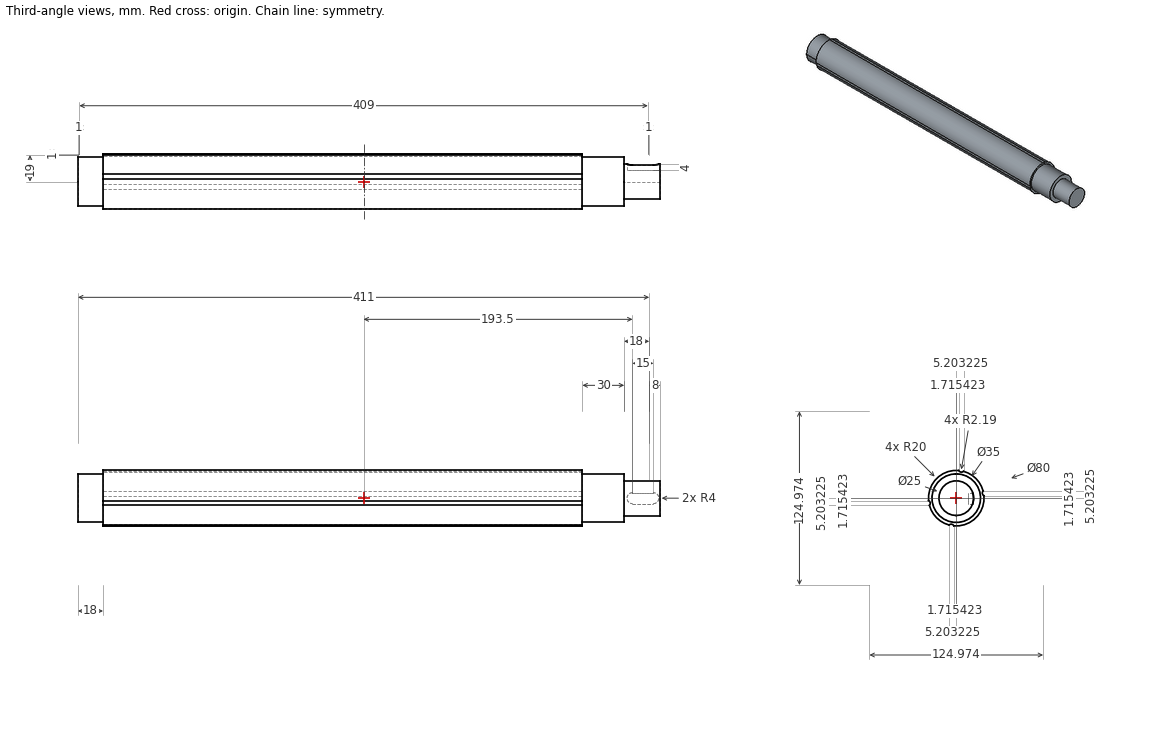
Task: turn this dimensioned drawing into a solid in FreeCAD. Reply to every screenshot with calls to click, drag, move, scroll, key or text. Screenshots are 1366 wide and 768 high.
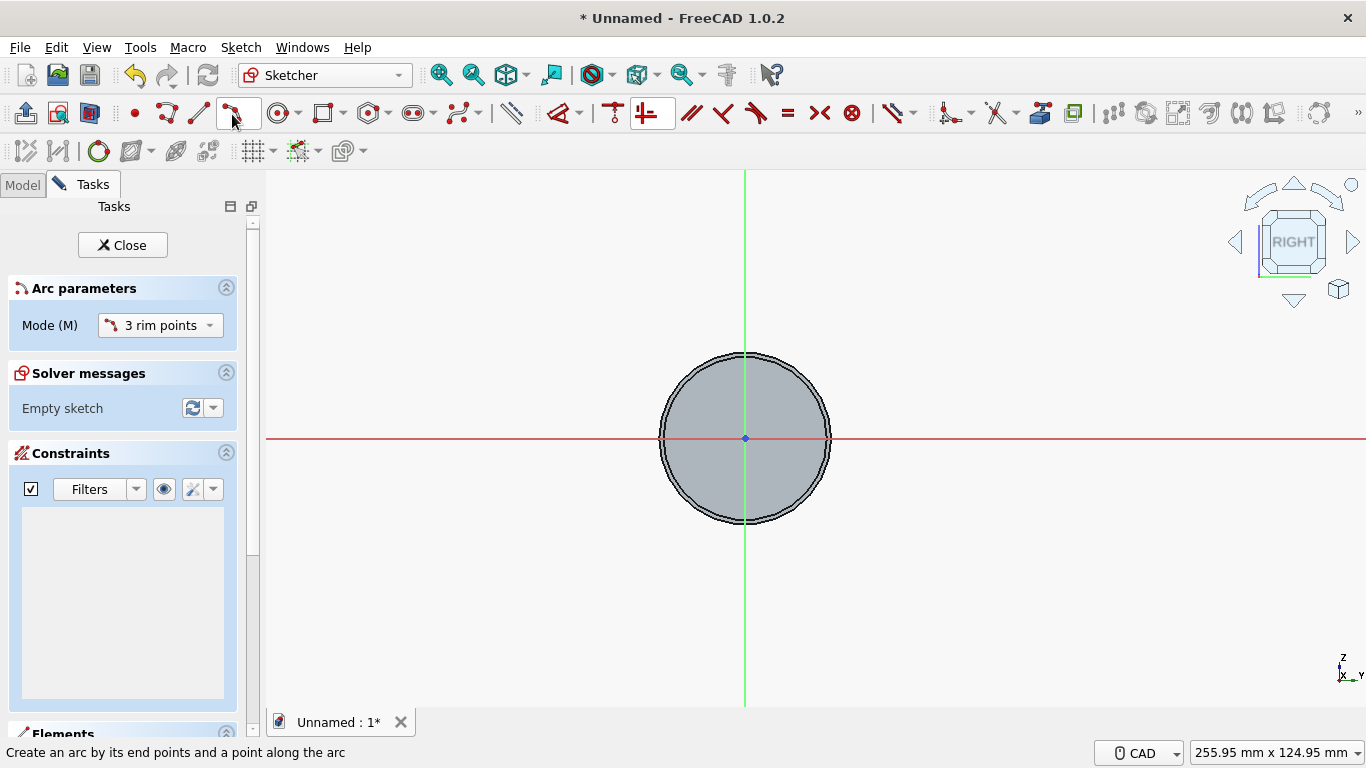
click(768, 356)
click(828, 416)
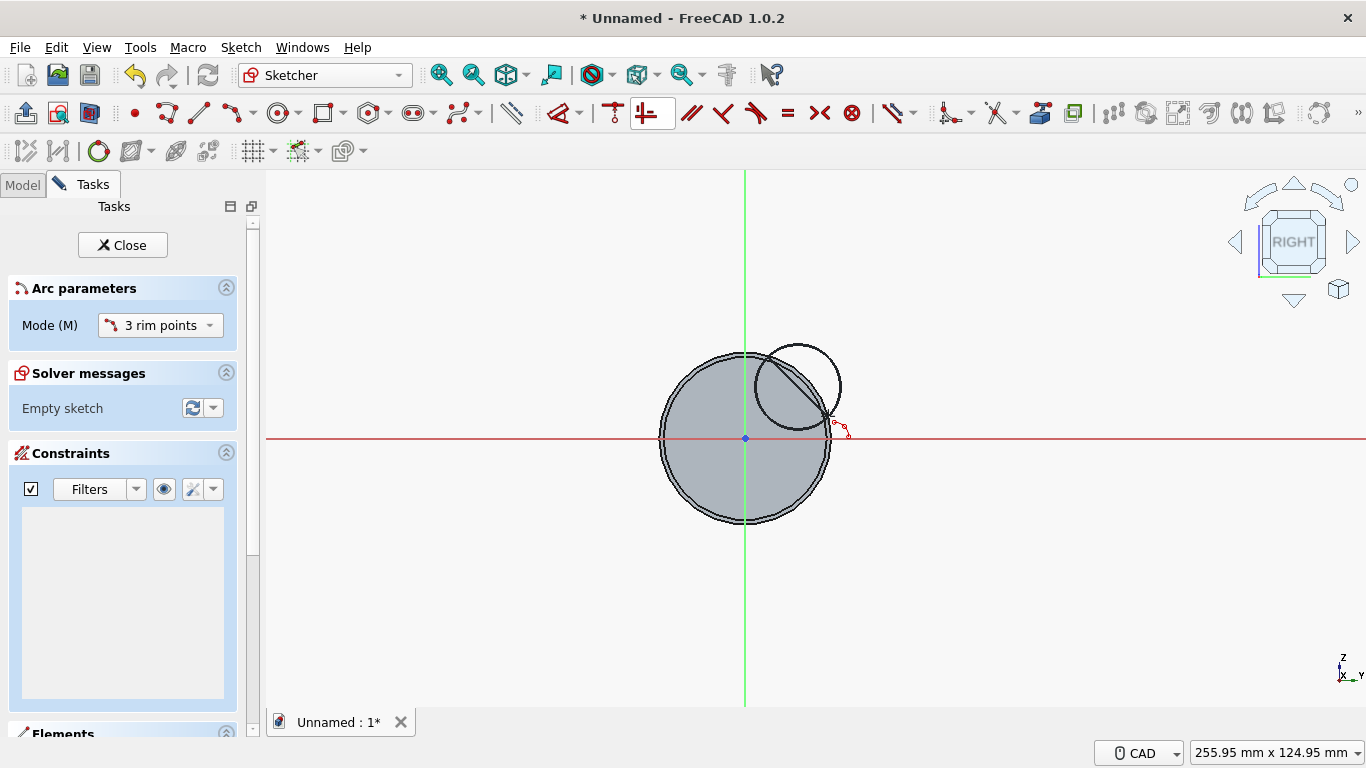
scroll(806, 378, up, 2)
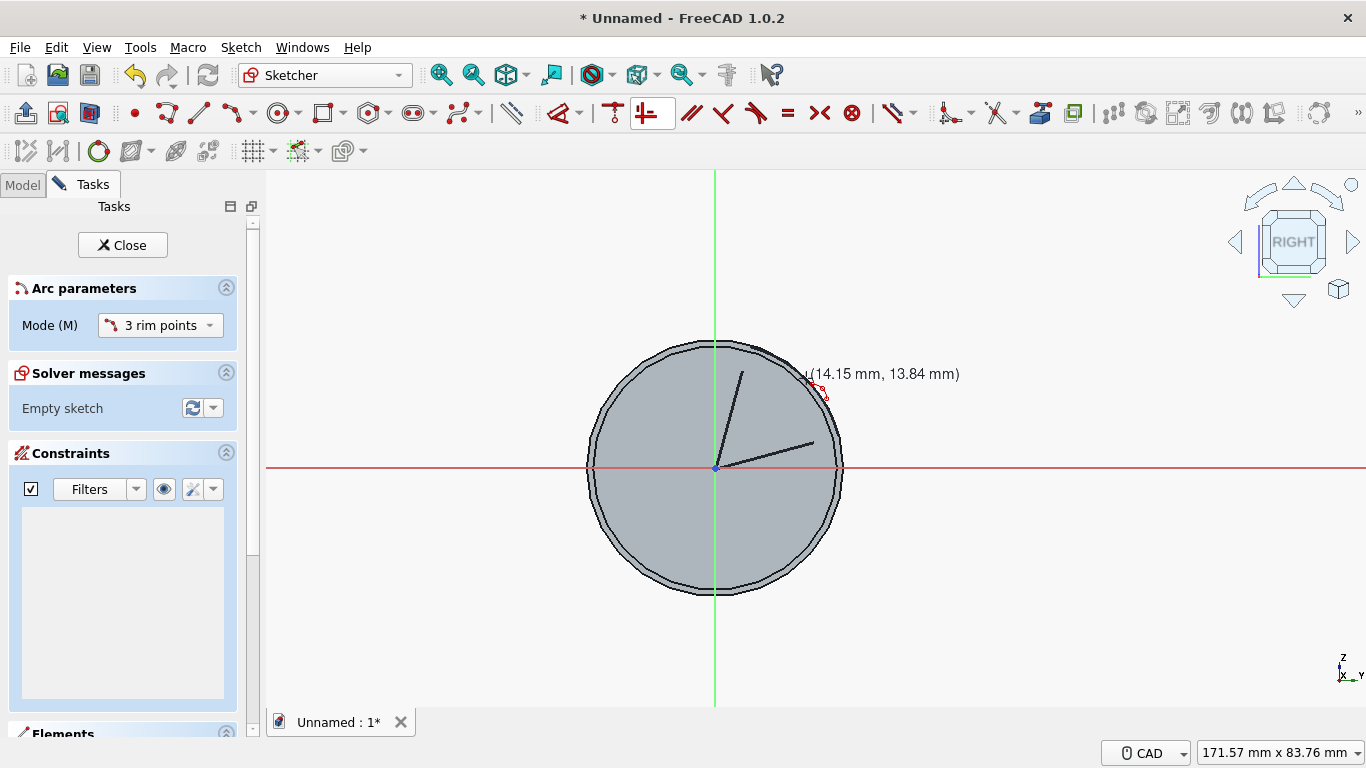
click(806, 377)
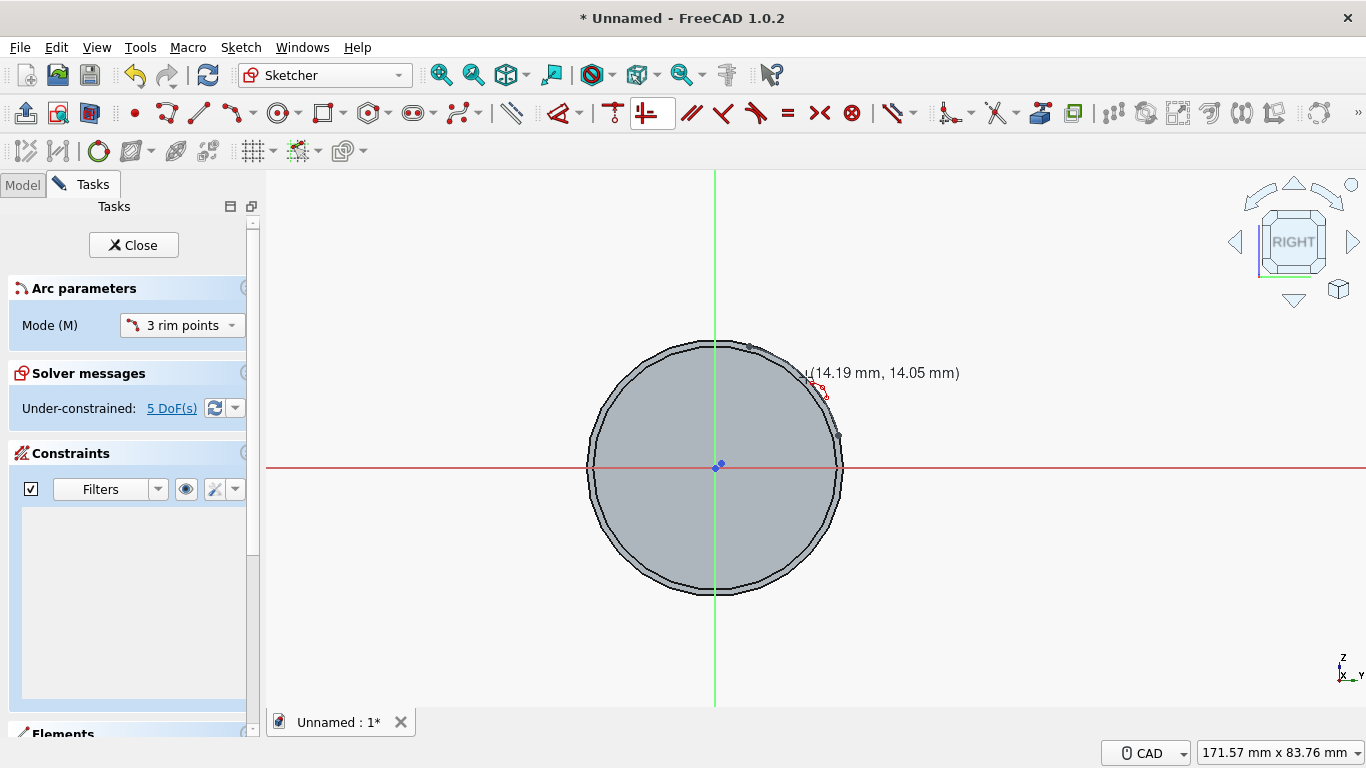
click(839, 436)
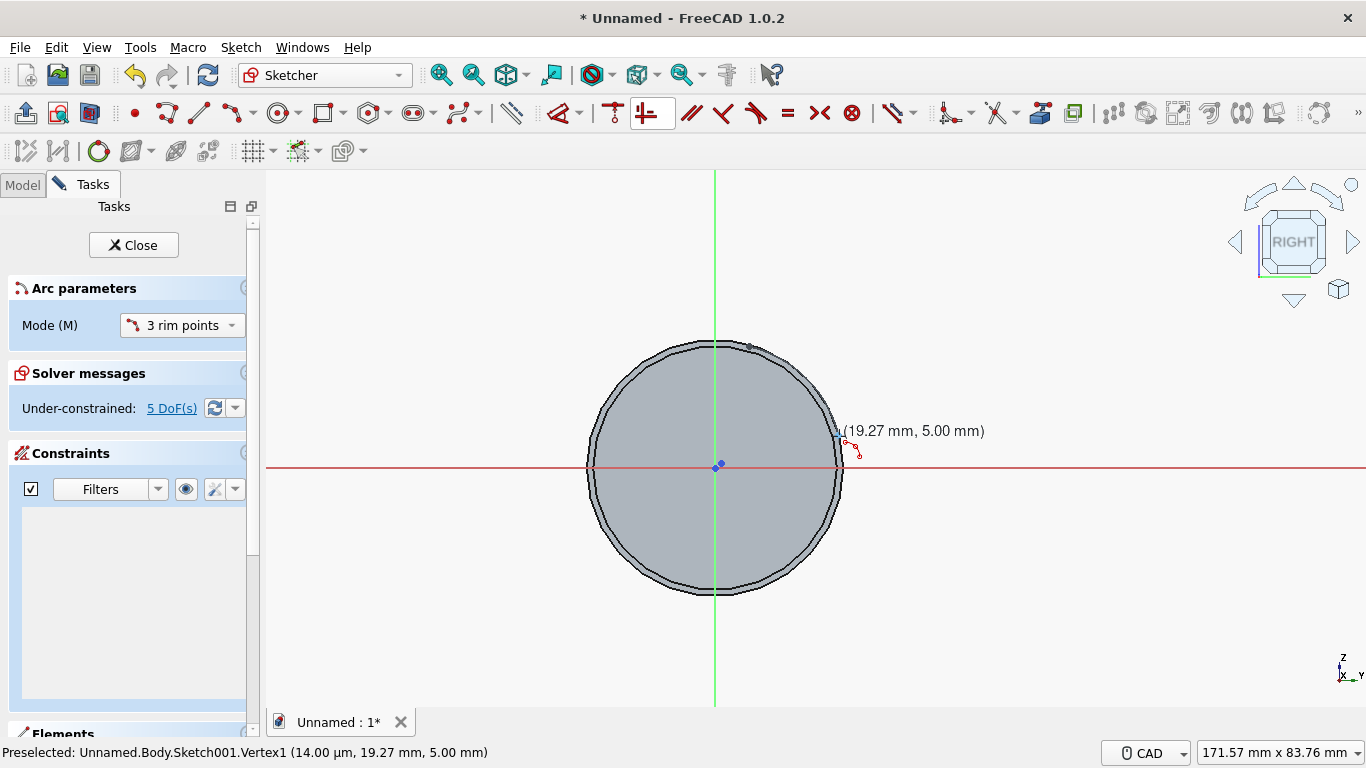
scroll(843, 457, up, 2)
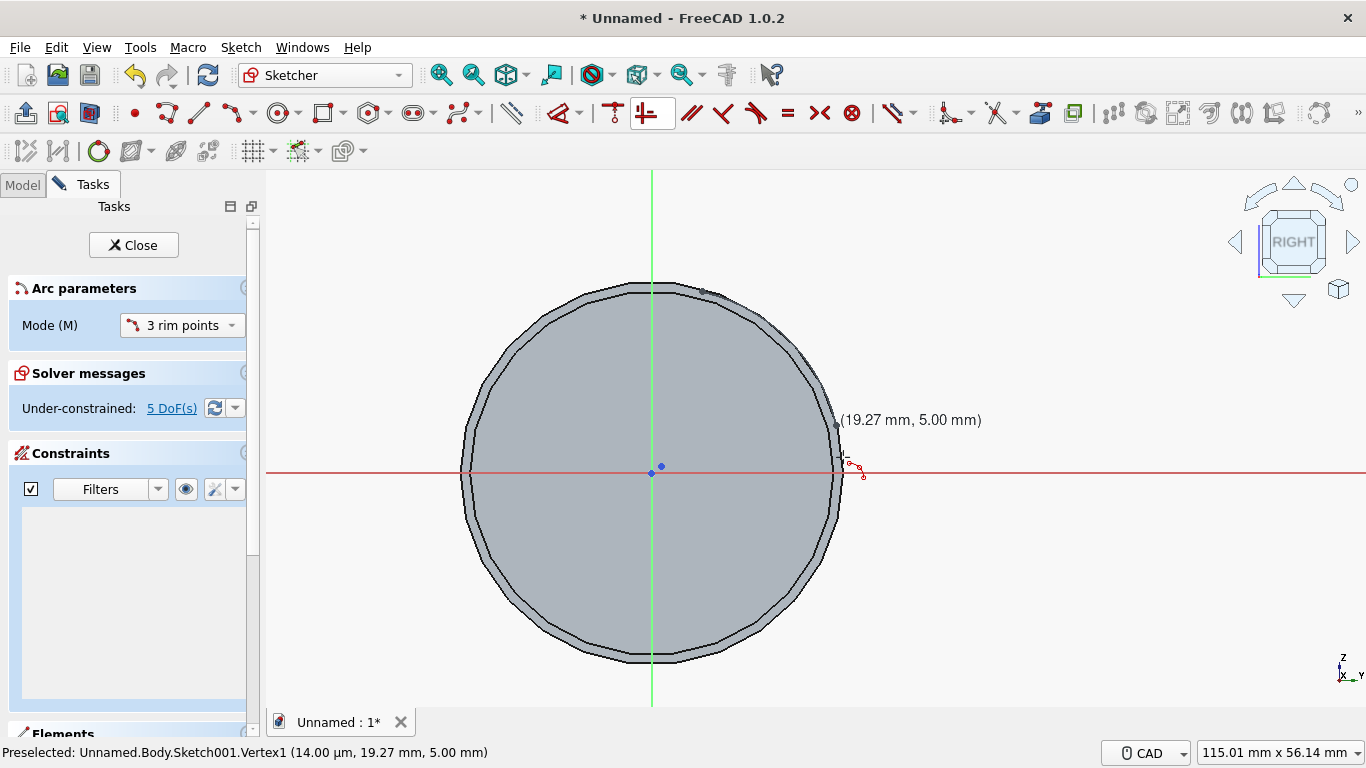
click(842, 457)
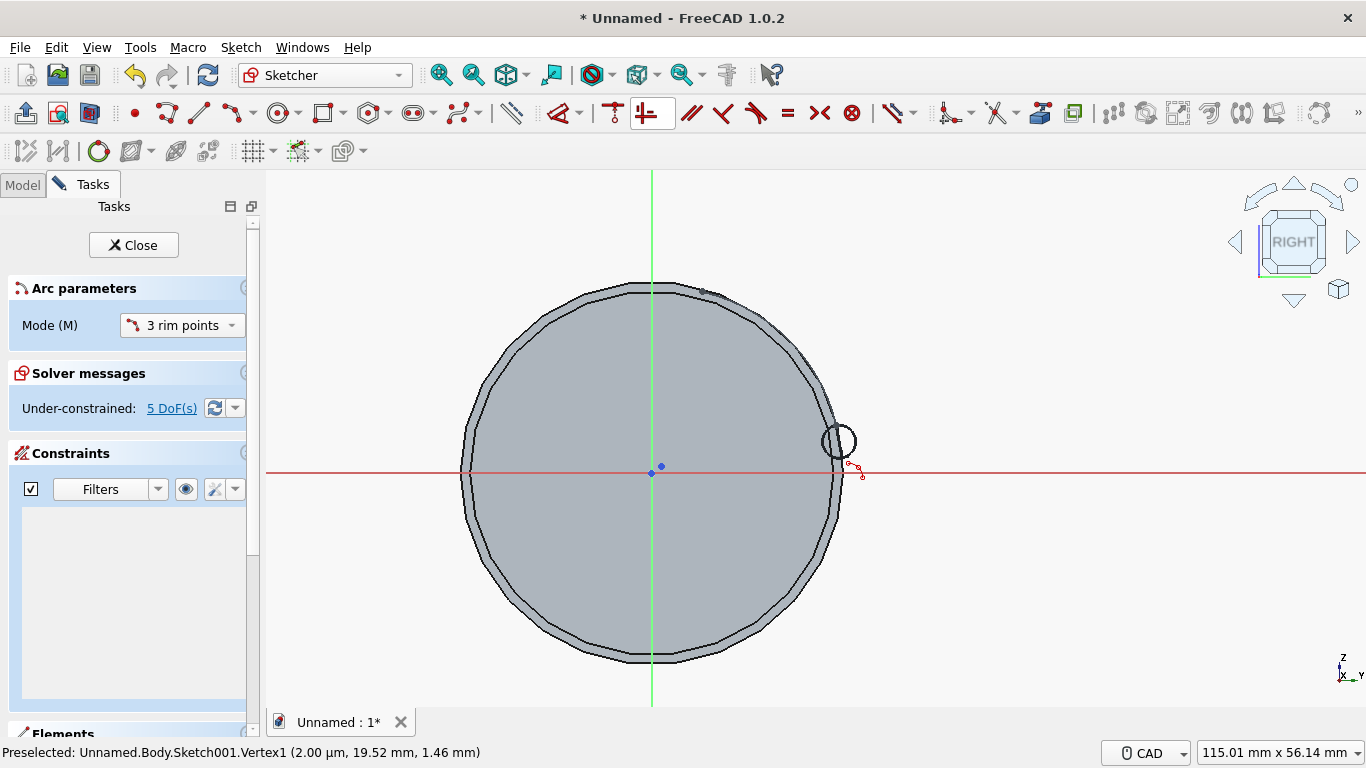
scroll(831, 442, up, 4)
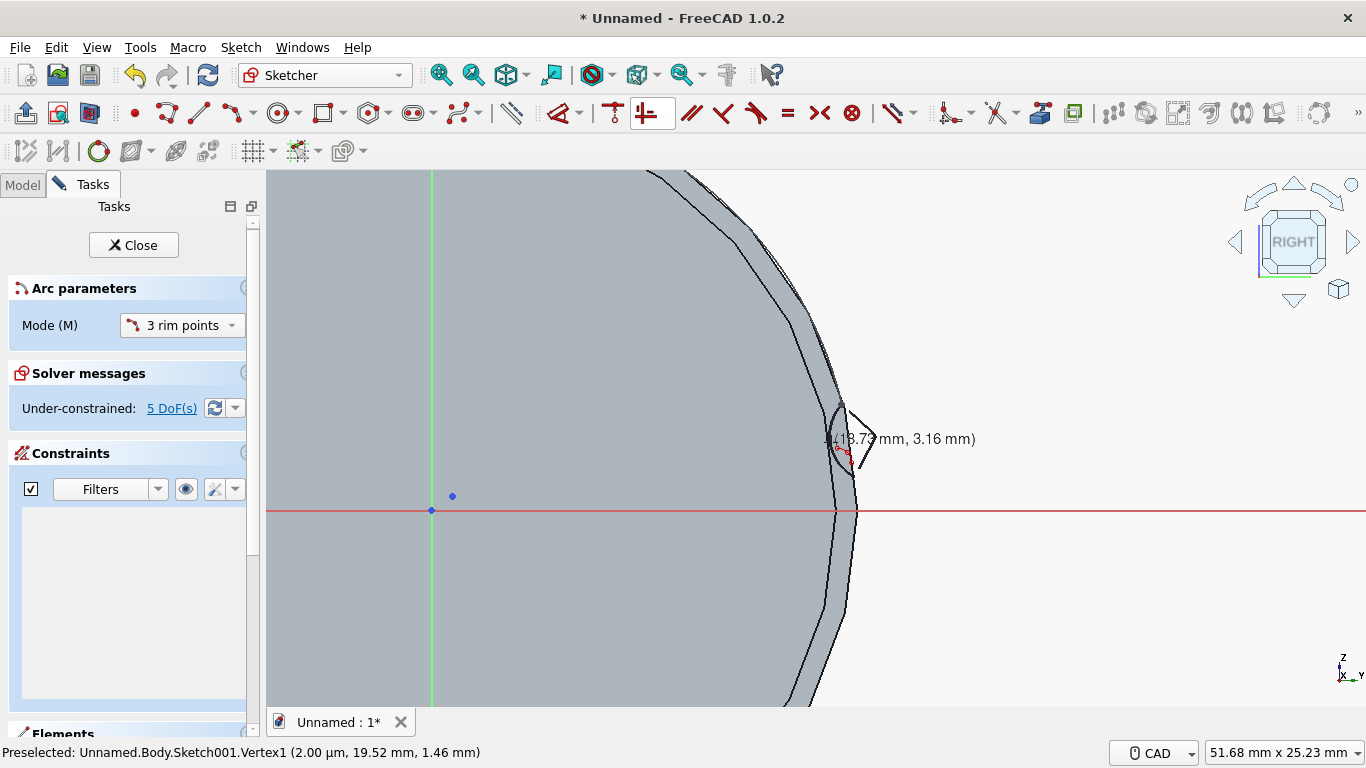
click(830, 441)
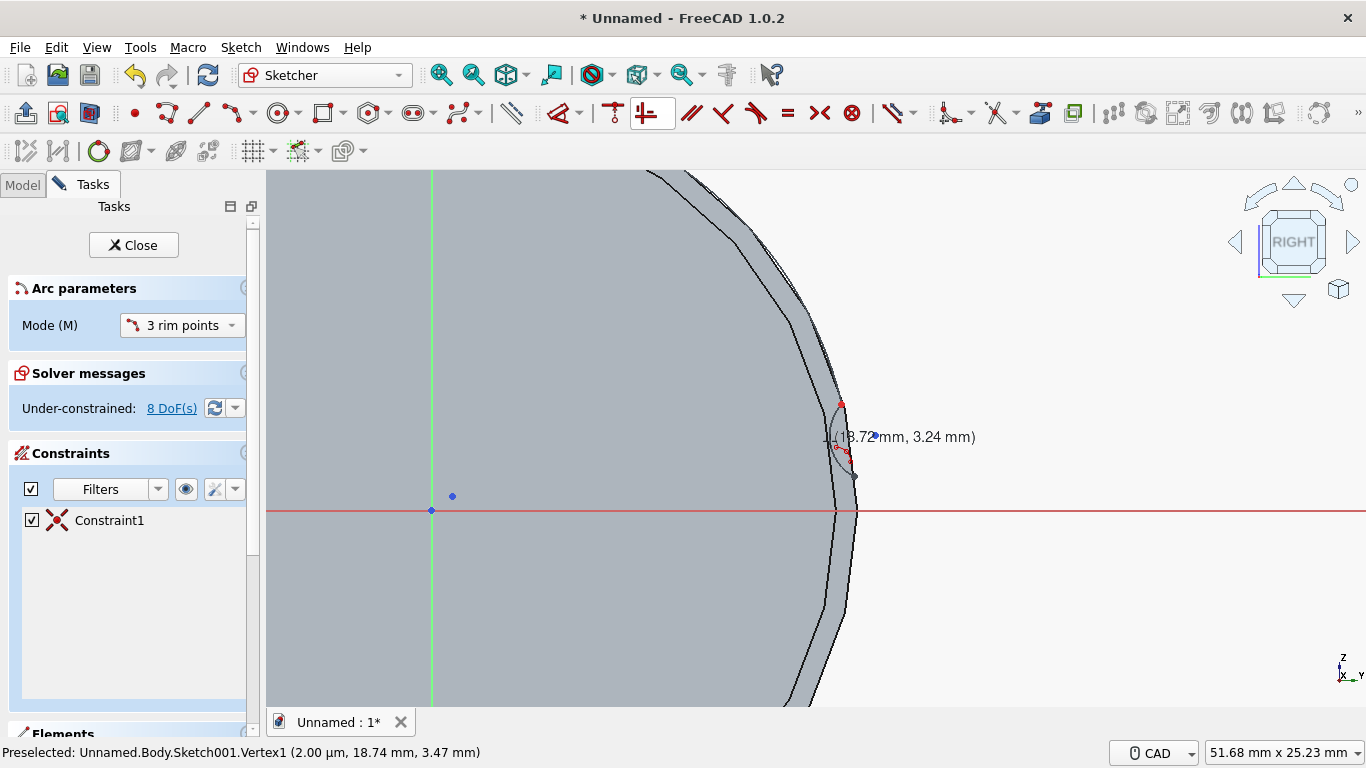
click(855, 477)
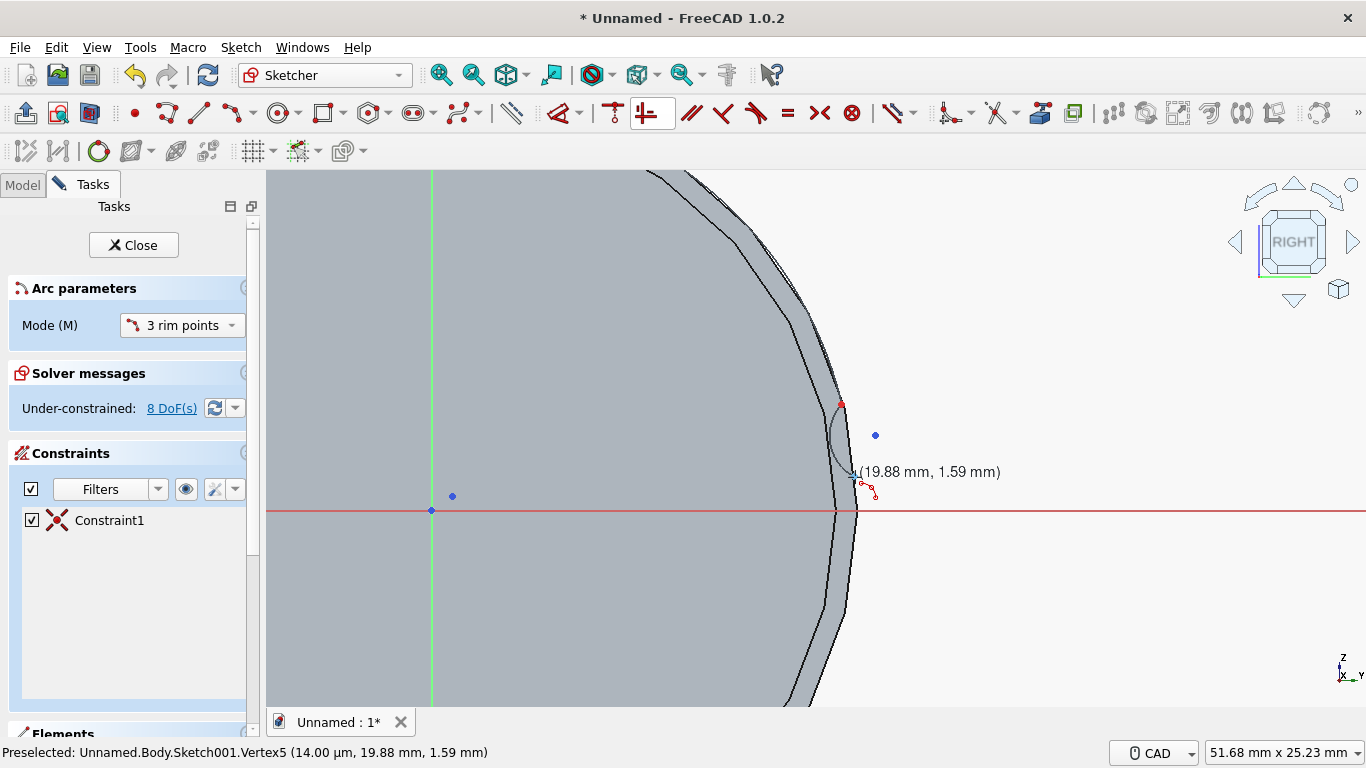
scroll(827, 420, down, 8)